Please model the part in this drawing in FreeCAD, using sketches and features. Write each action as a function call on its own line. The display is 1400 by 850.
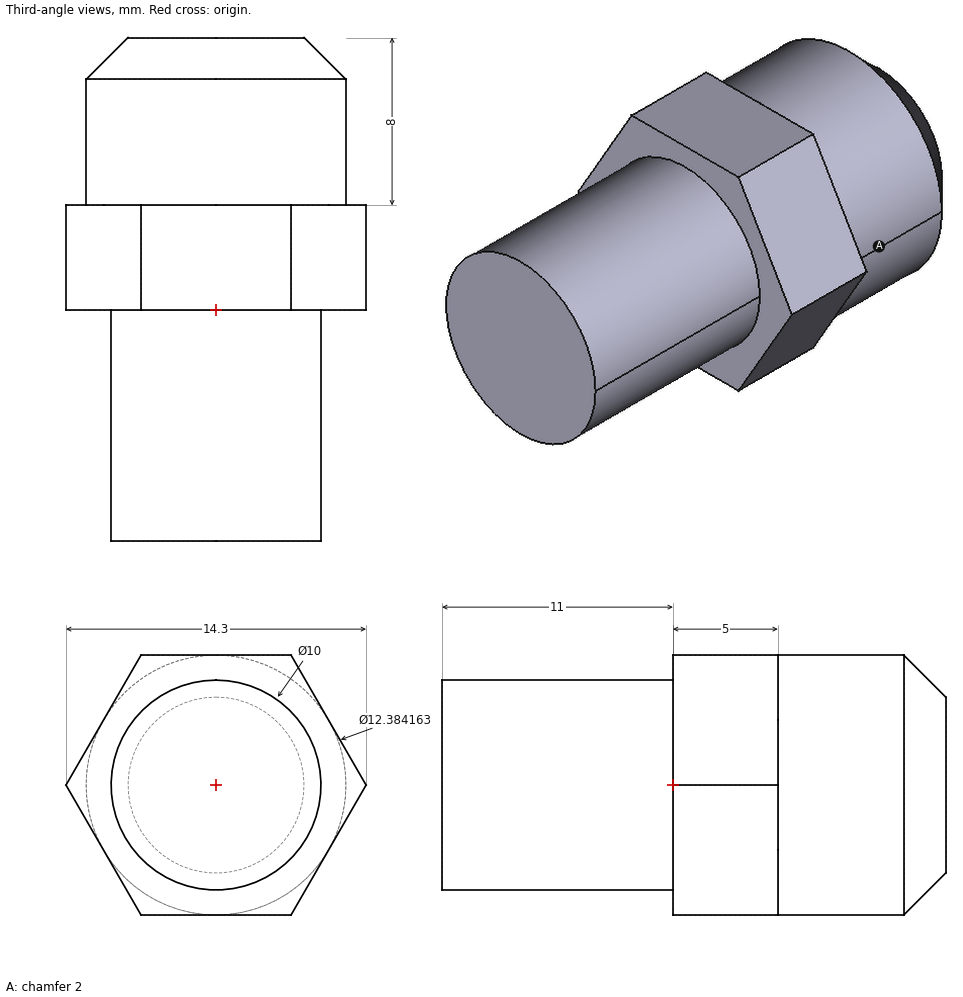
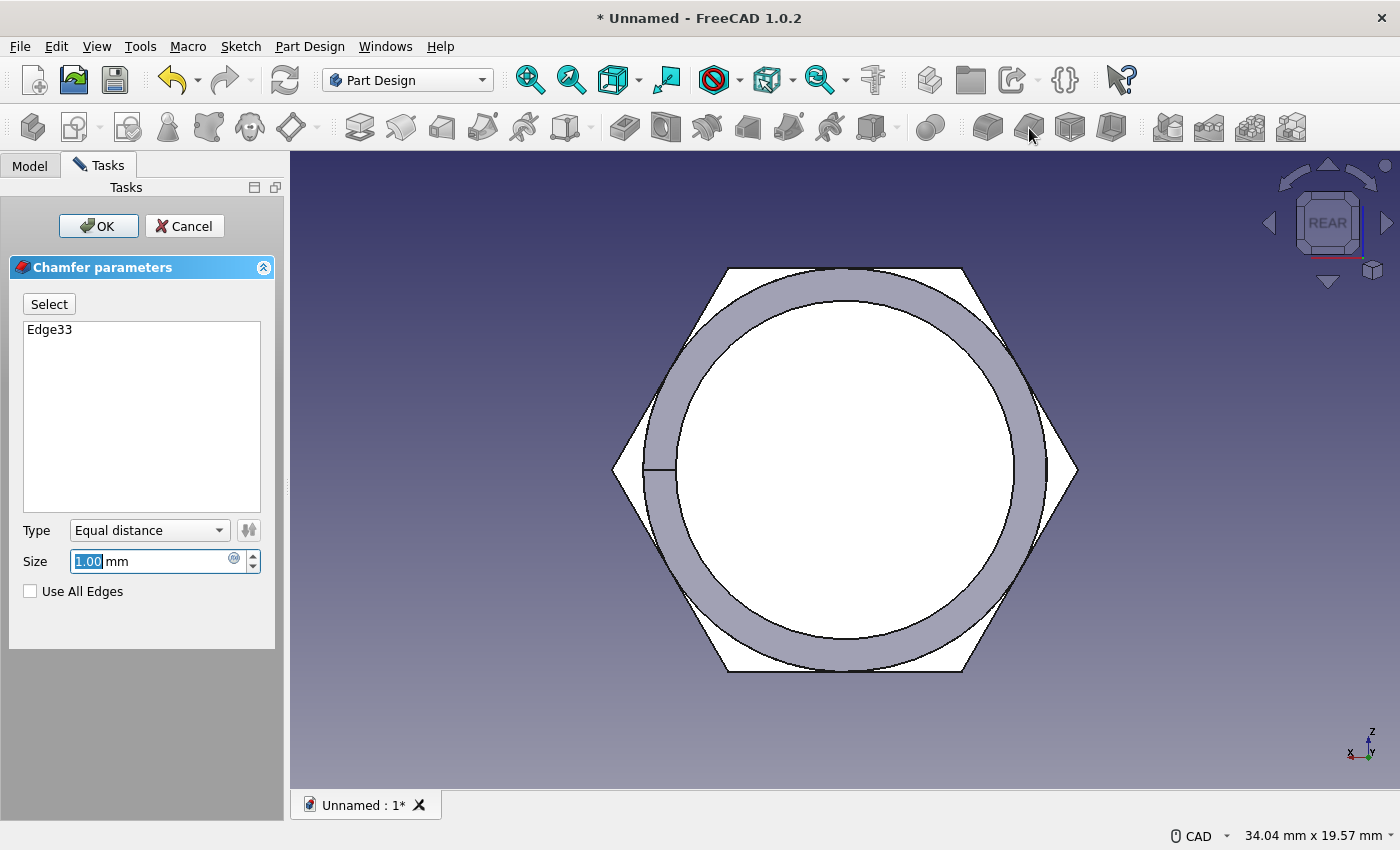
text(2)
key(Tab)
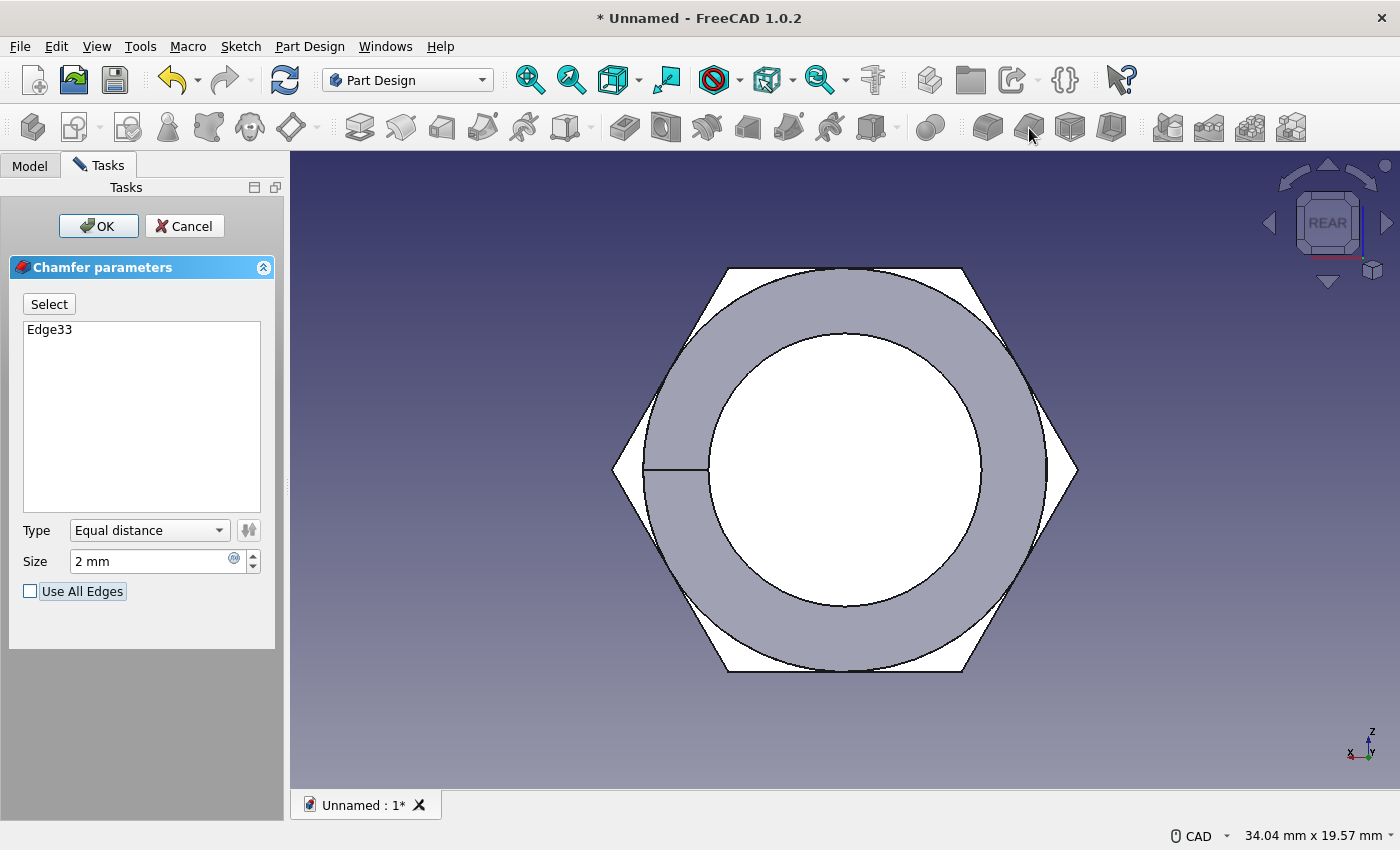
click(99, 226)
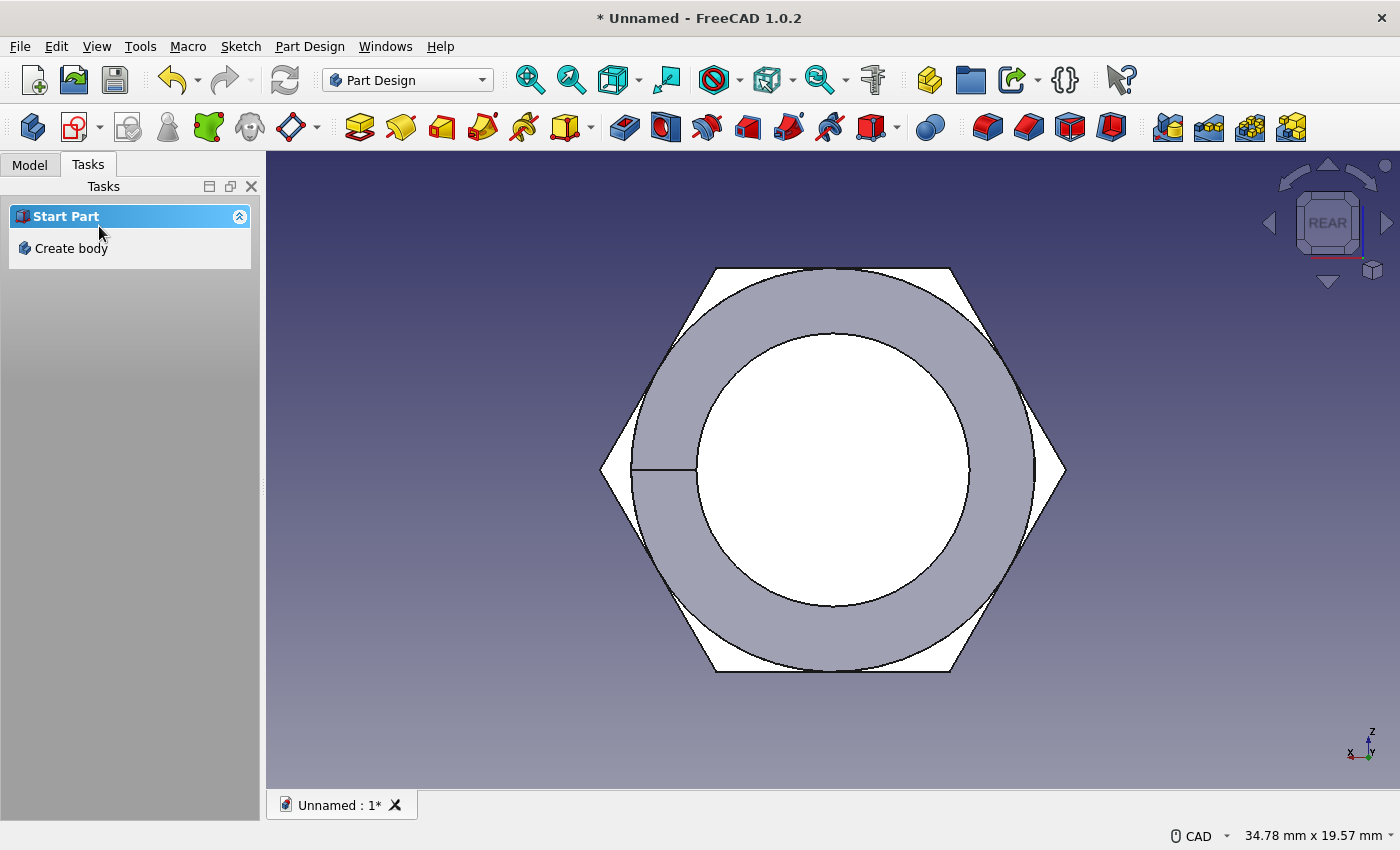
click(74, 128)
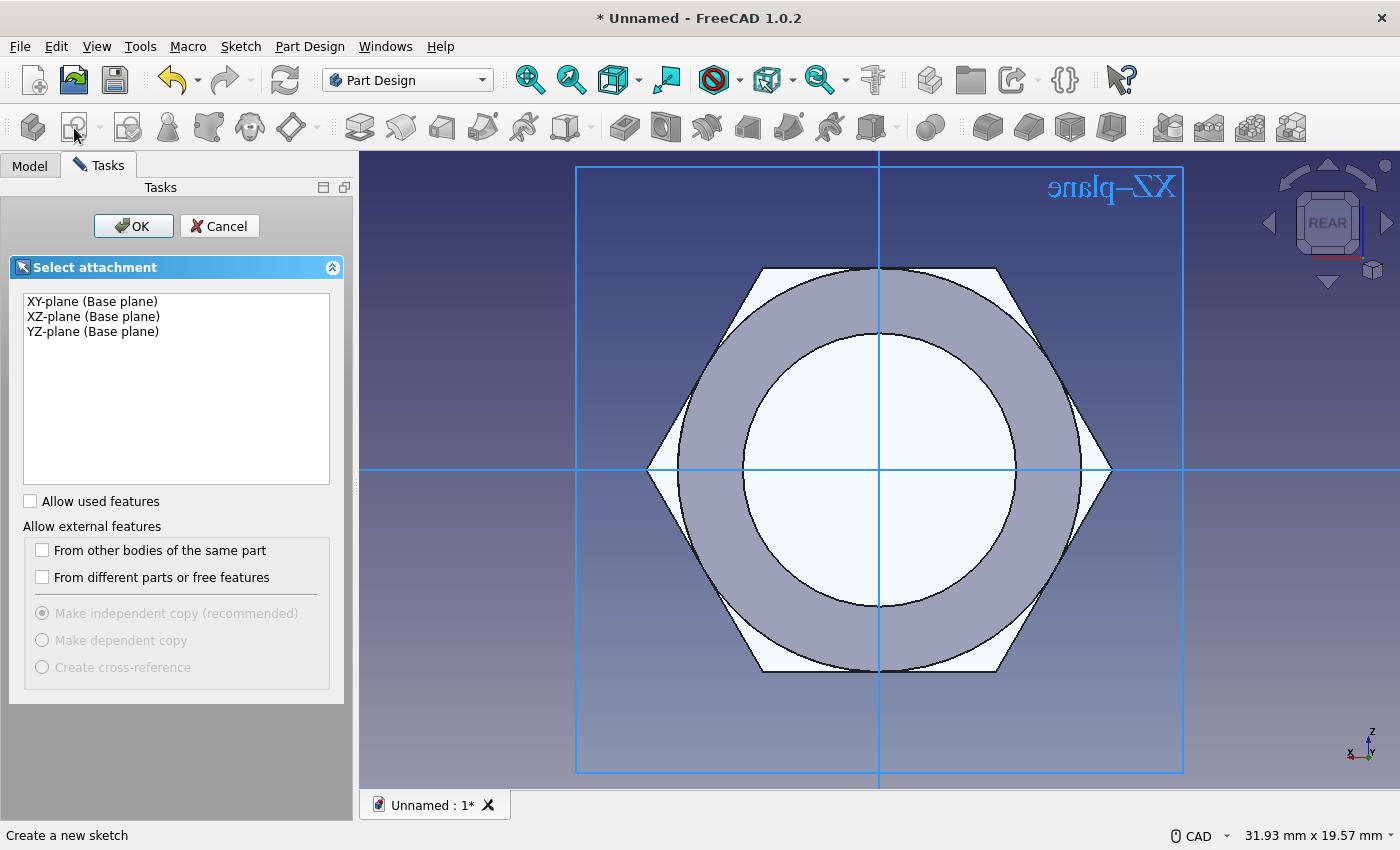
click(84, 316)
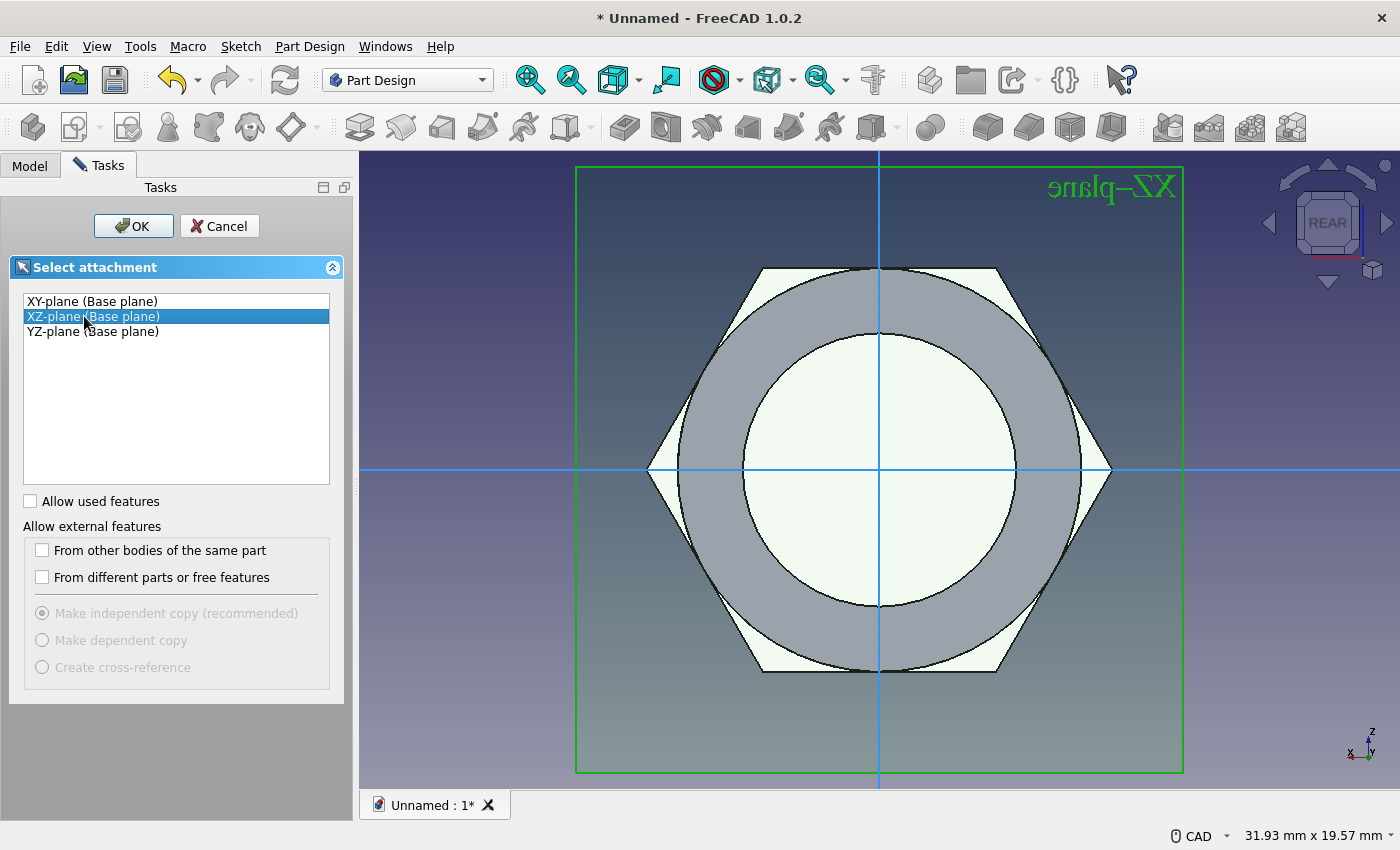
click(134, 226)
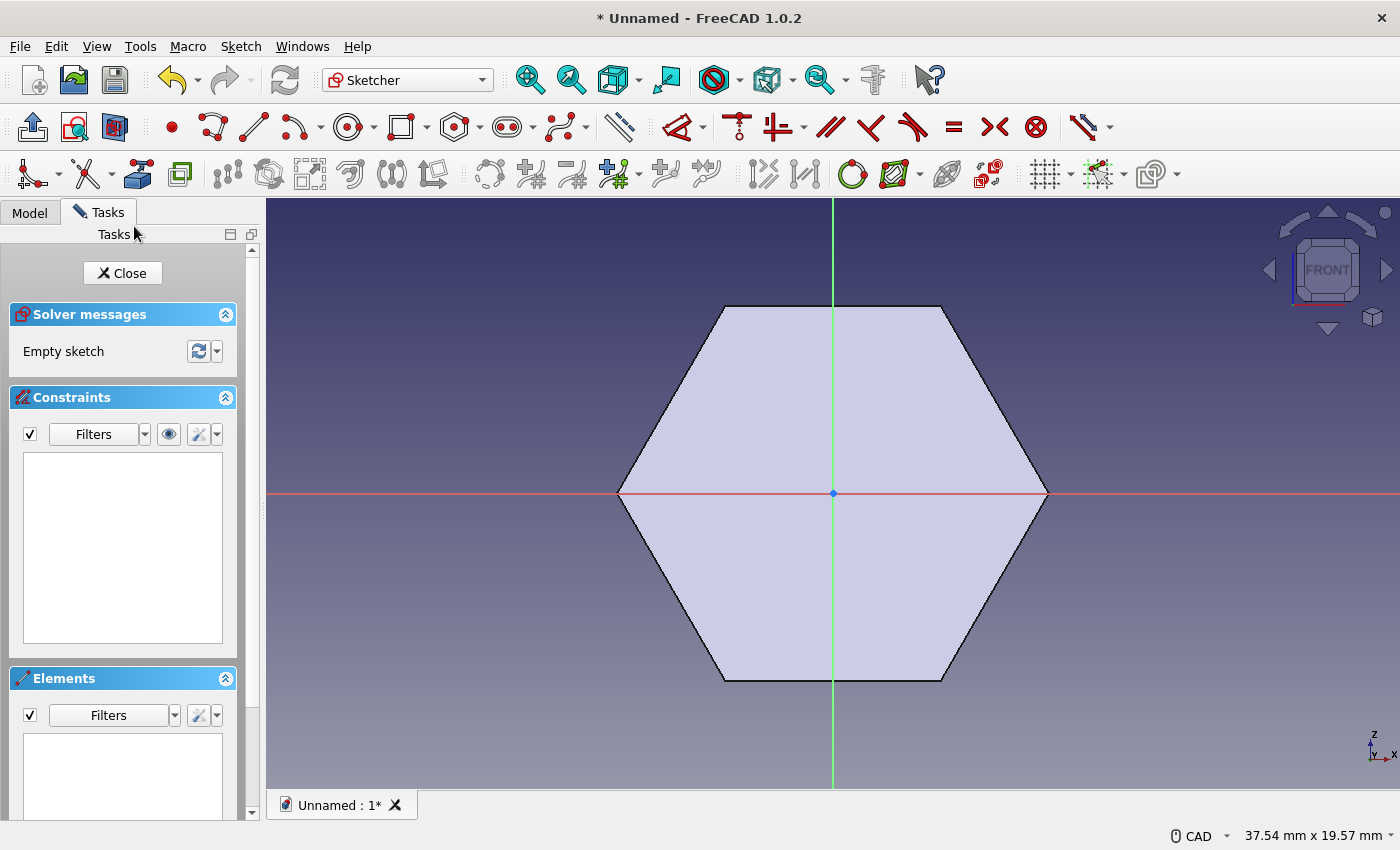
click(348, 128)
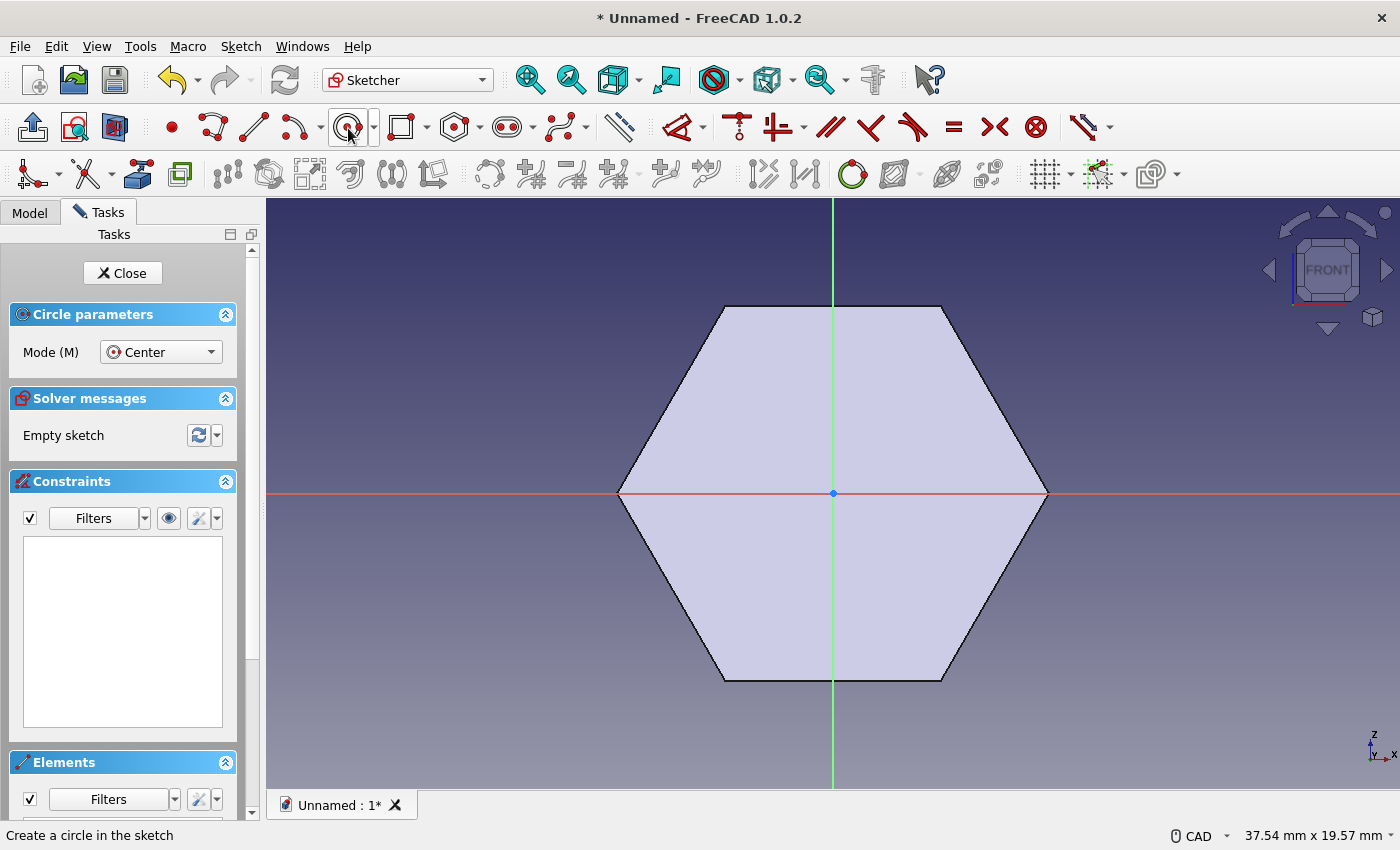
click(833, 494)
click(940, 387)
key(Escape)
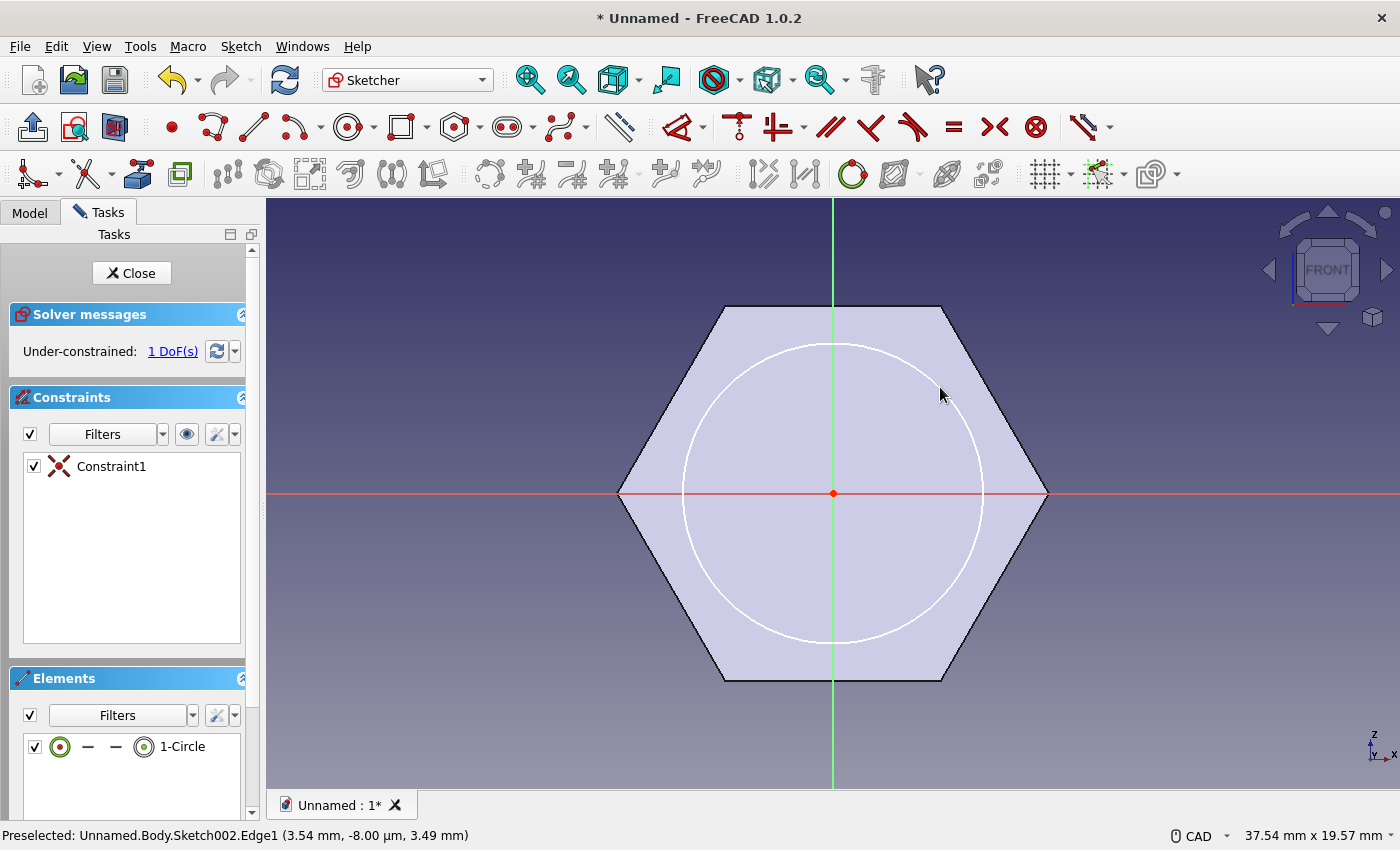
click(676, 128)